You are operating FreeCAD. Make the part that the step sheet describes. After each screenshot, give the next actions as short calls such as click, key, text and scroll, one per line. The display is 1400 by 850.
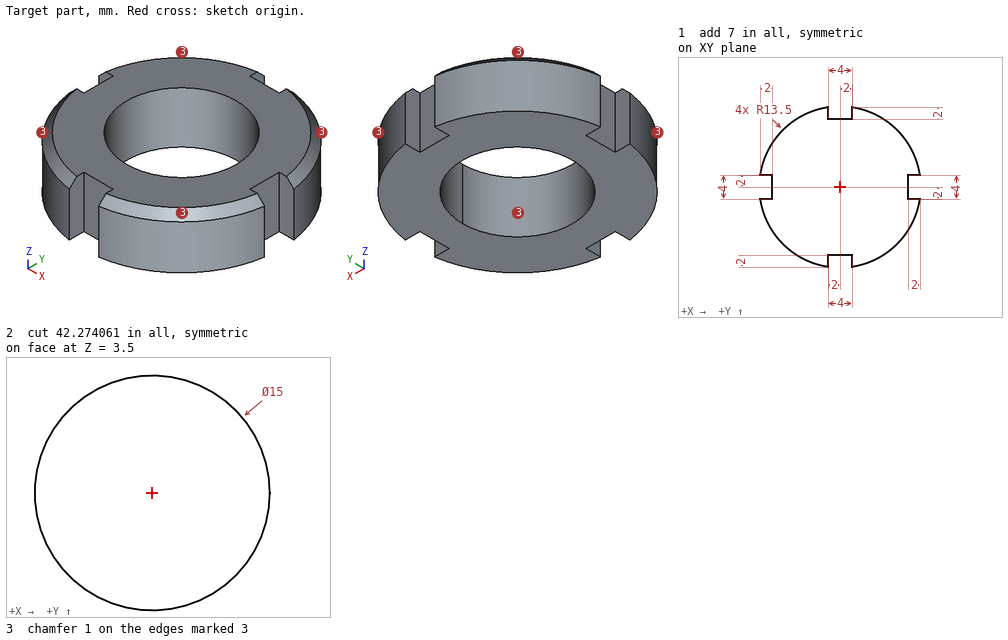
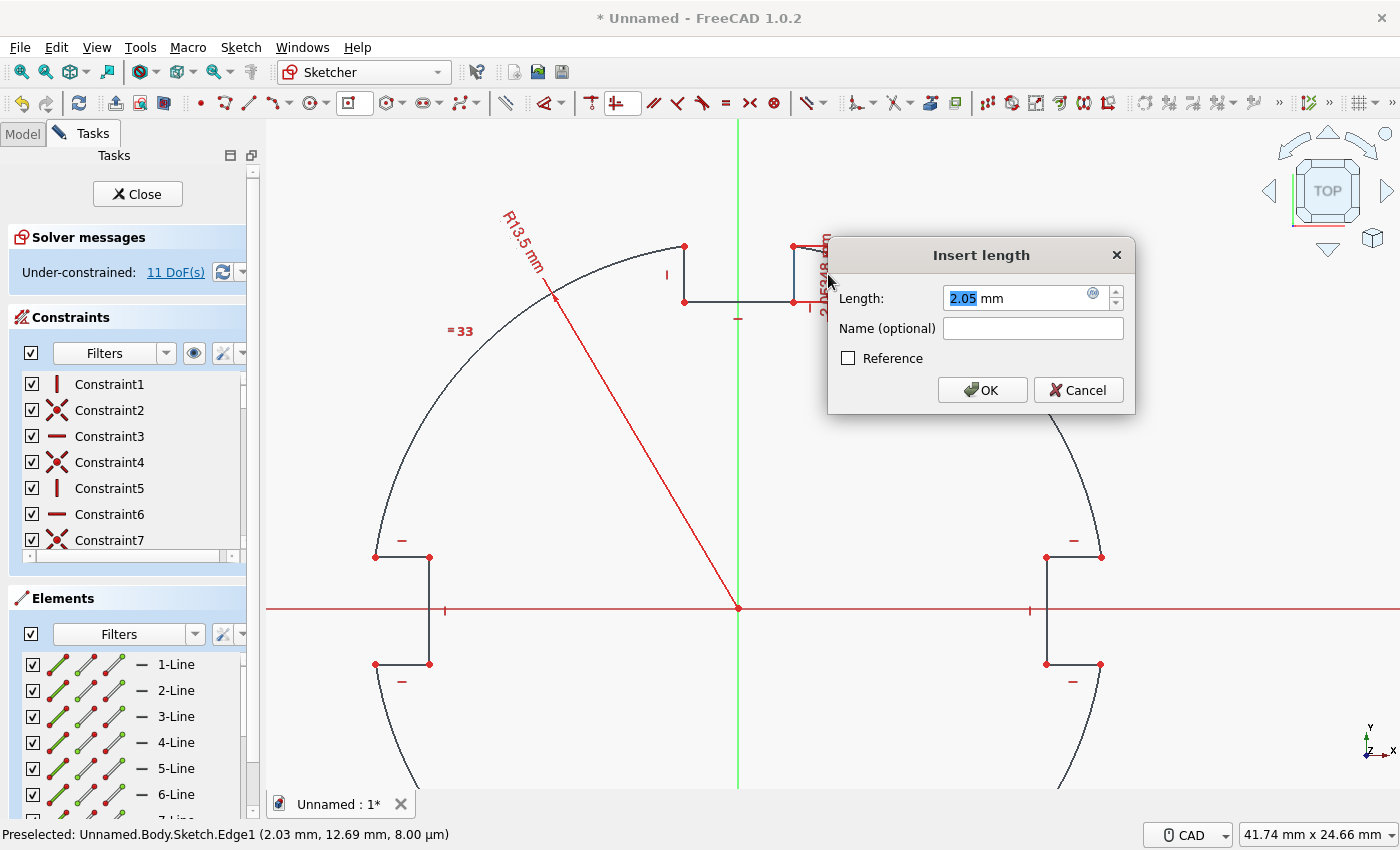
text(2)
key(Return)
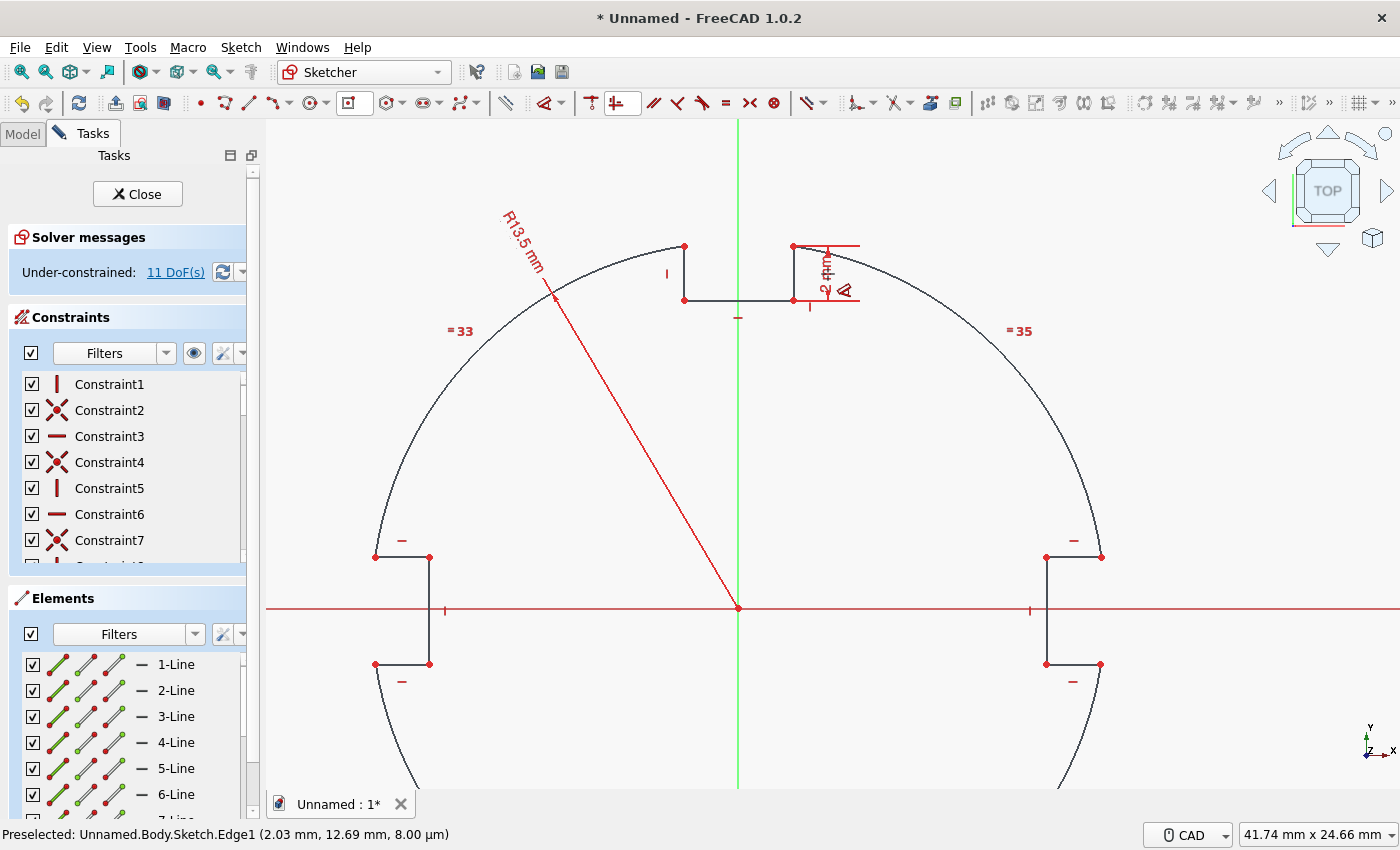
click(761, 301)
click(714, 267)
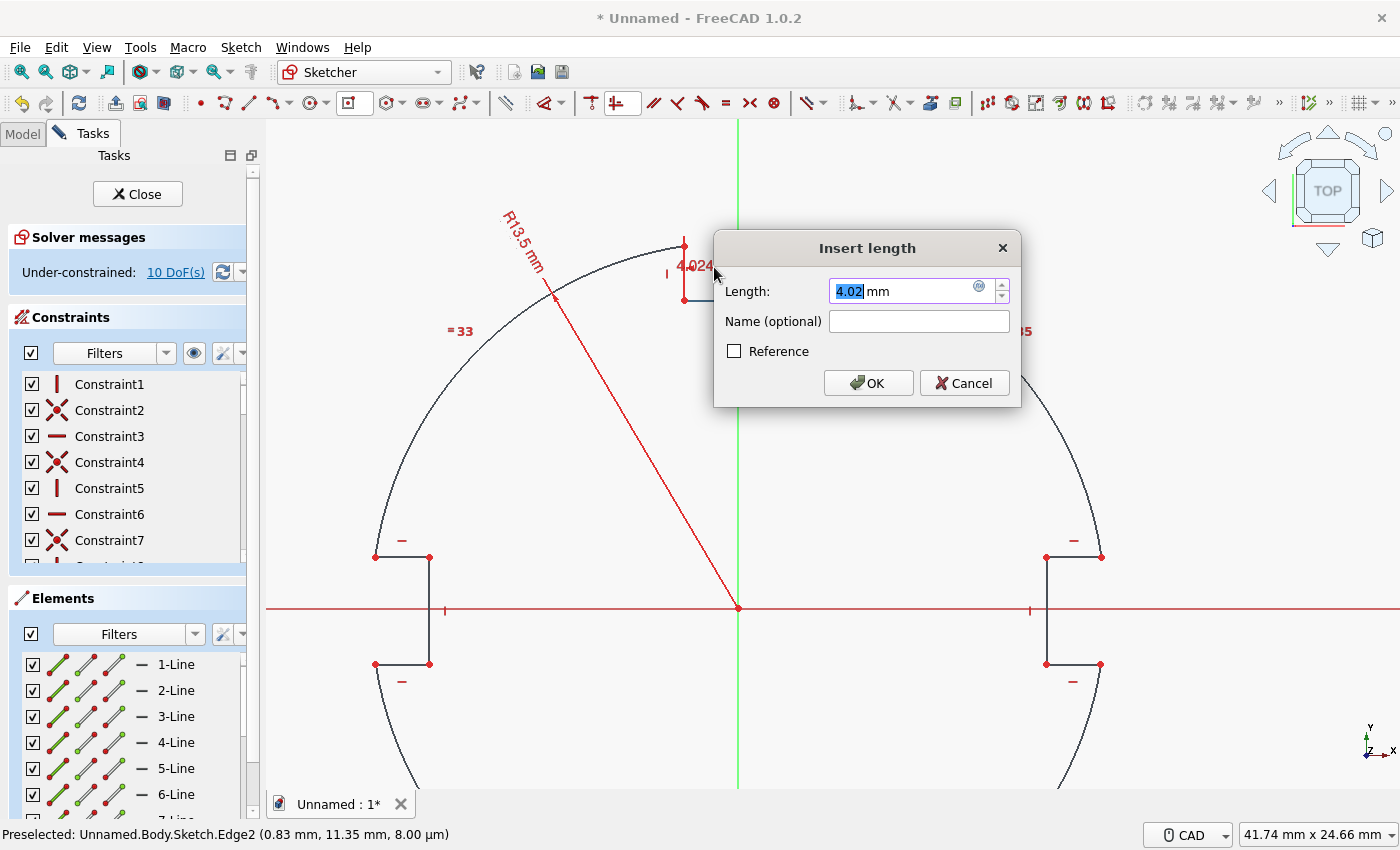
text(4)
key(Return)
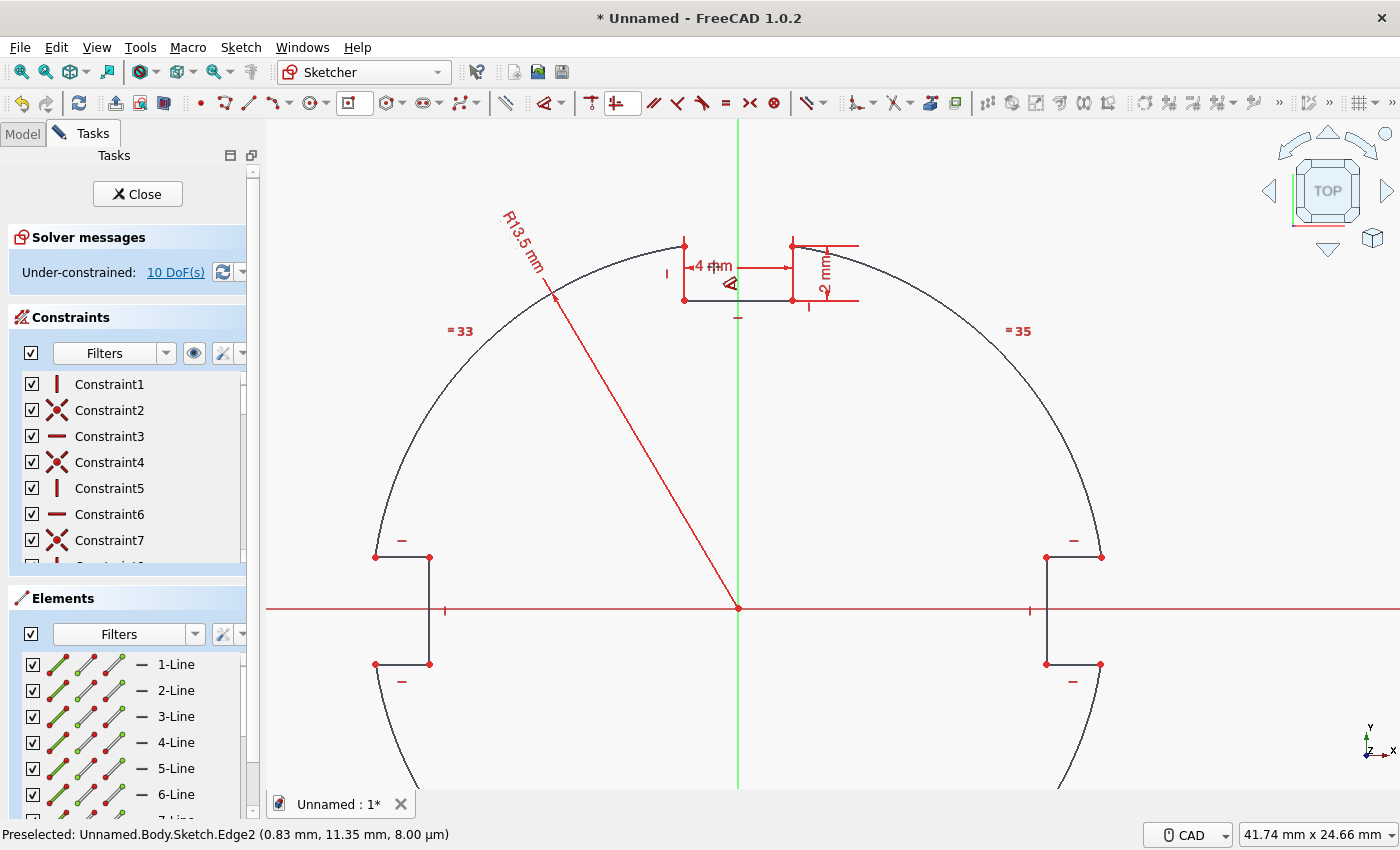
click(391, 557)
click(402, 523)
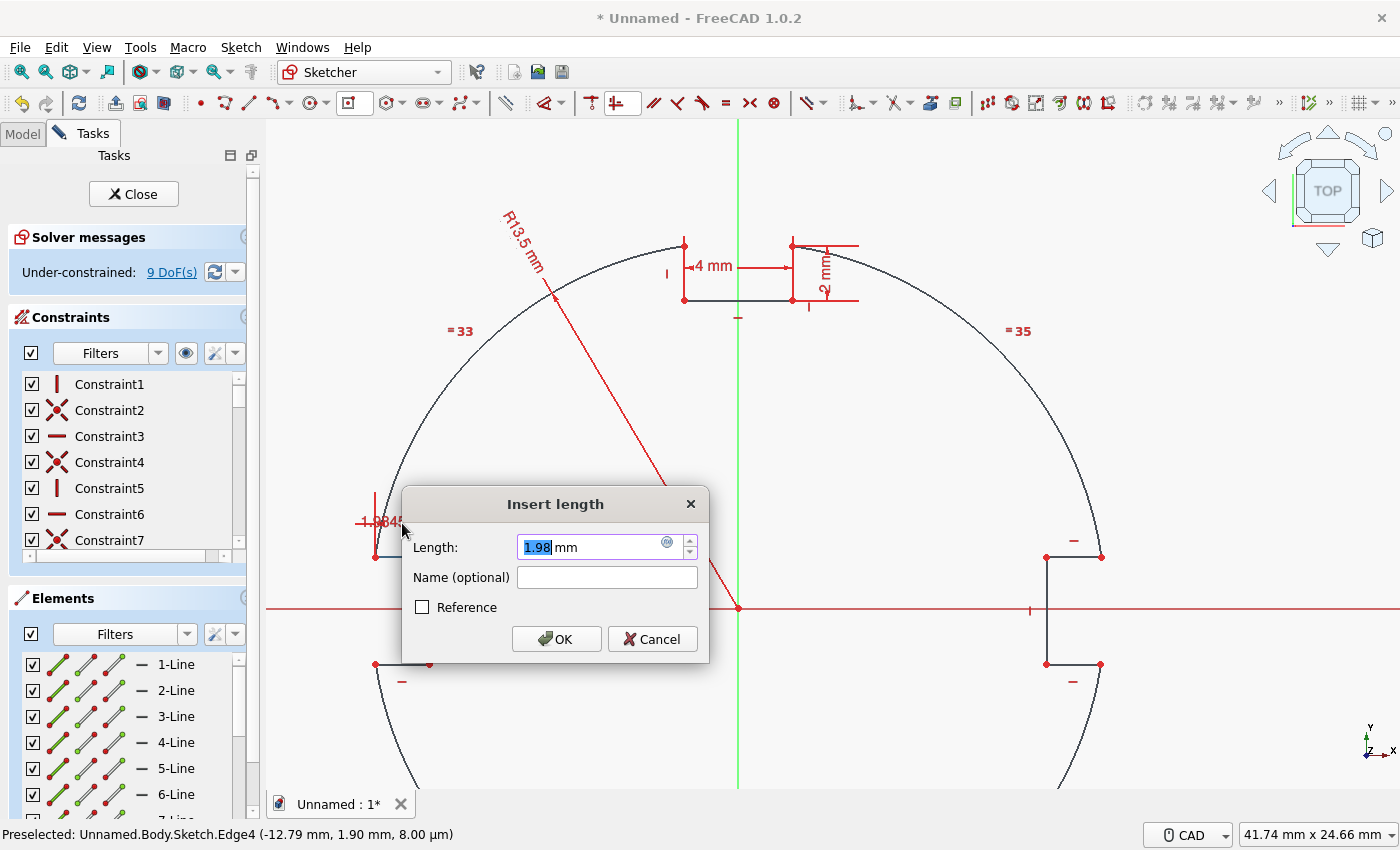
text(2)
key(Return)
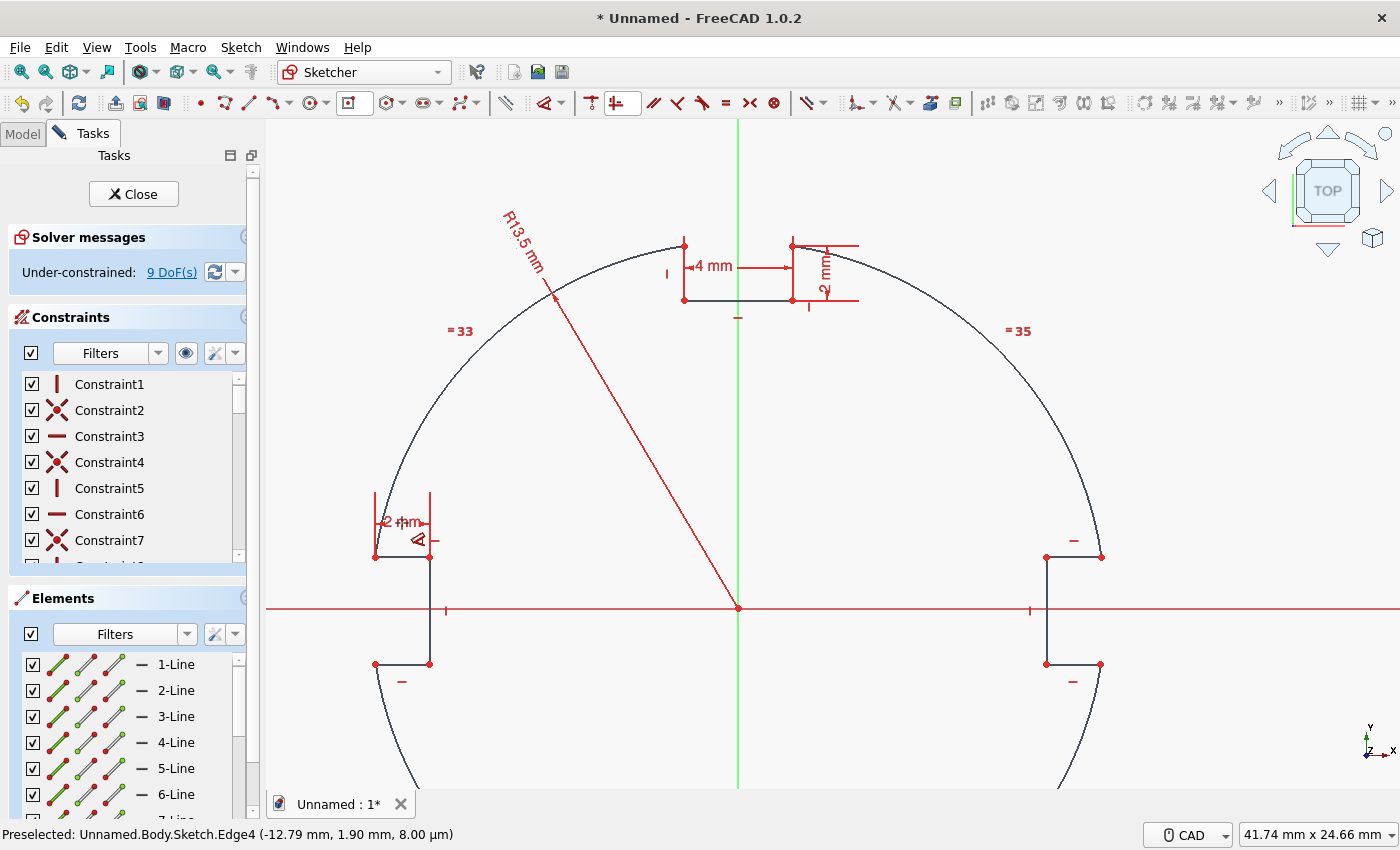
click(430, 589)
click(396, 586)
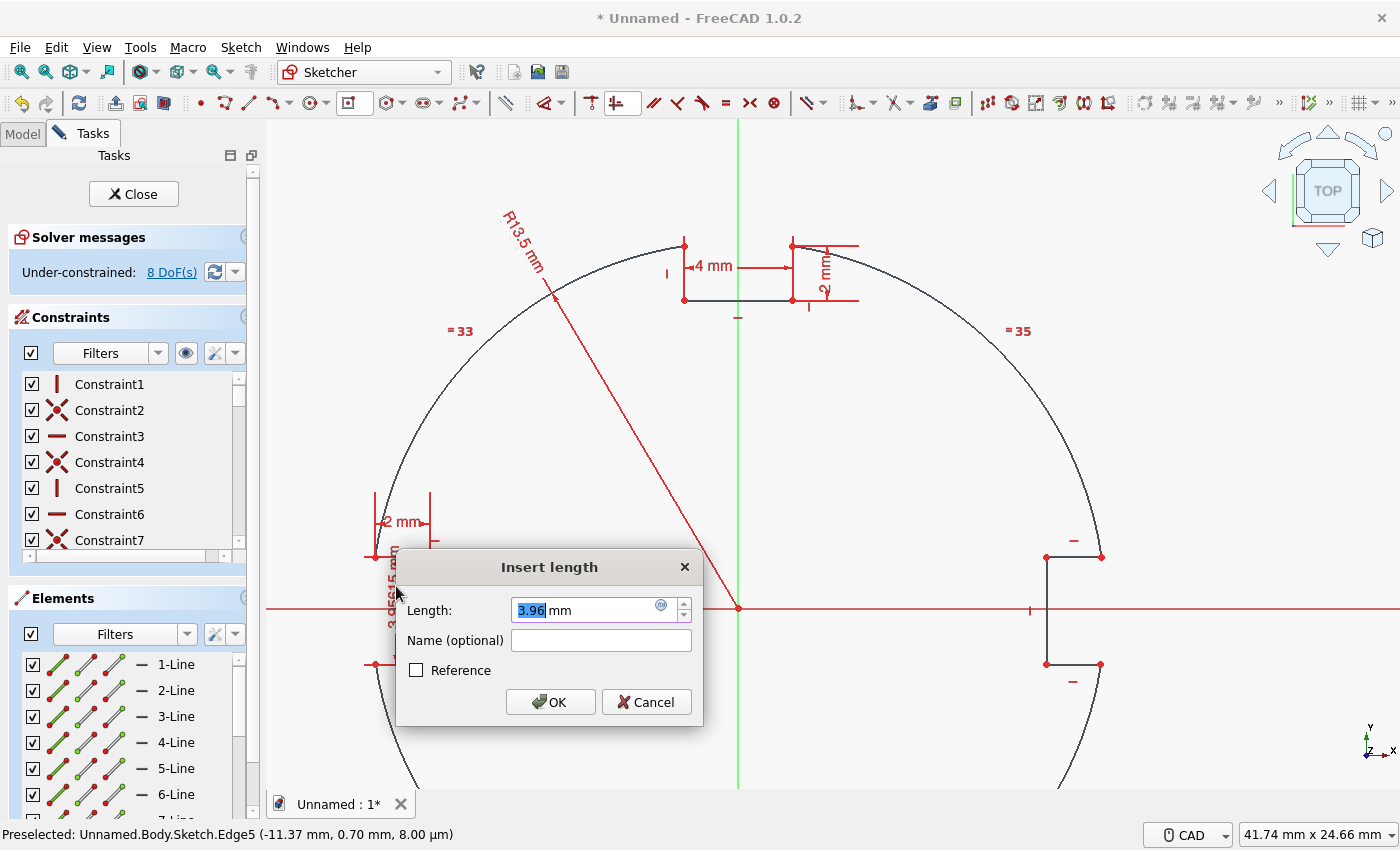
text(4)
key(Return)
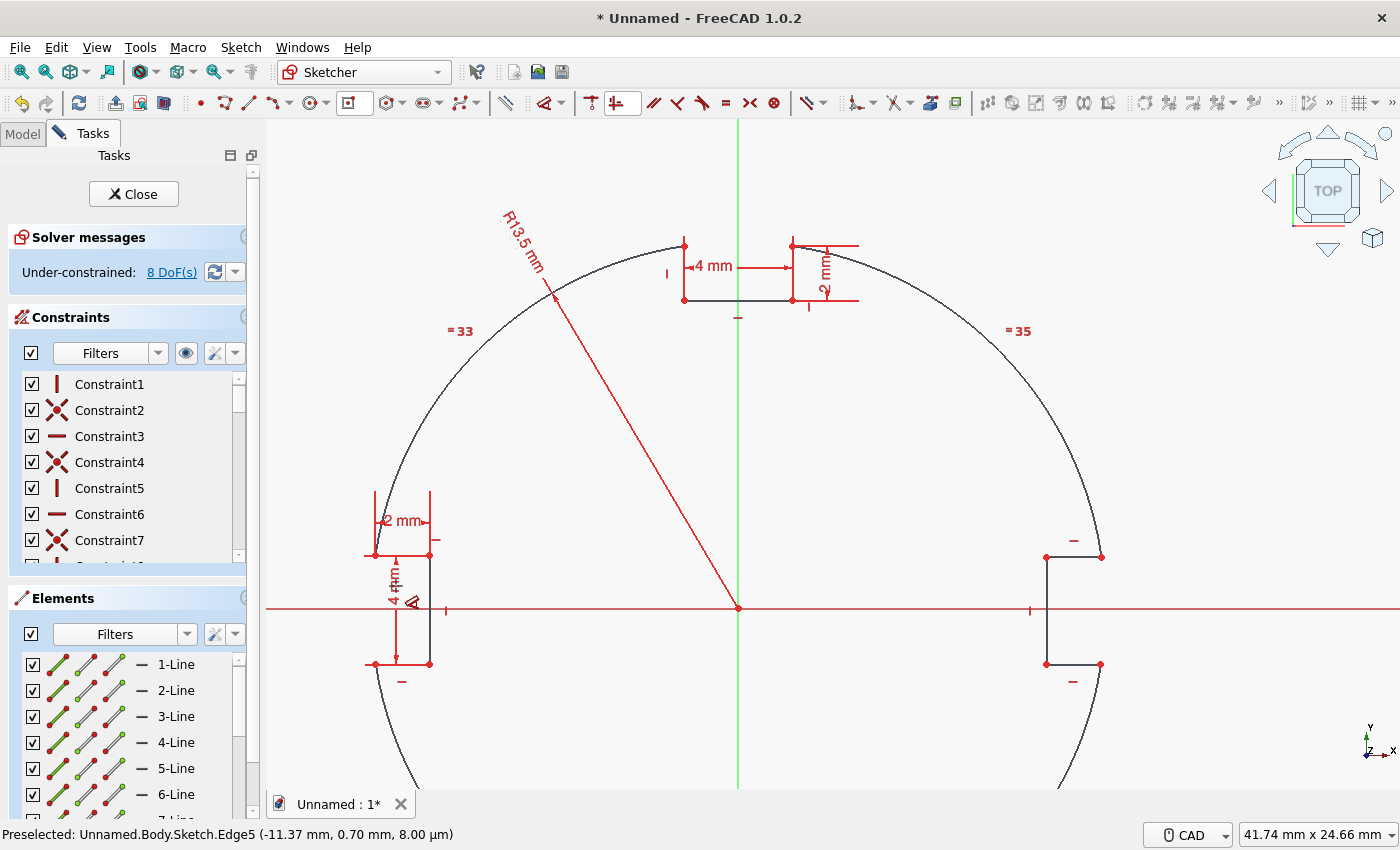
scroll(796, 266, down, 3)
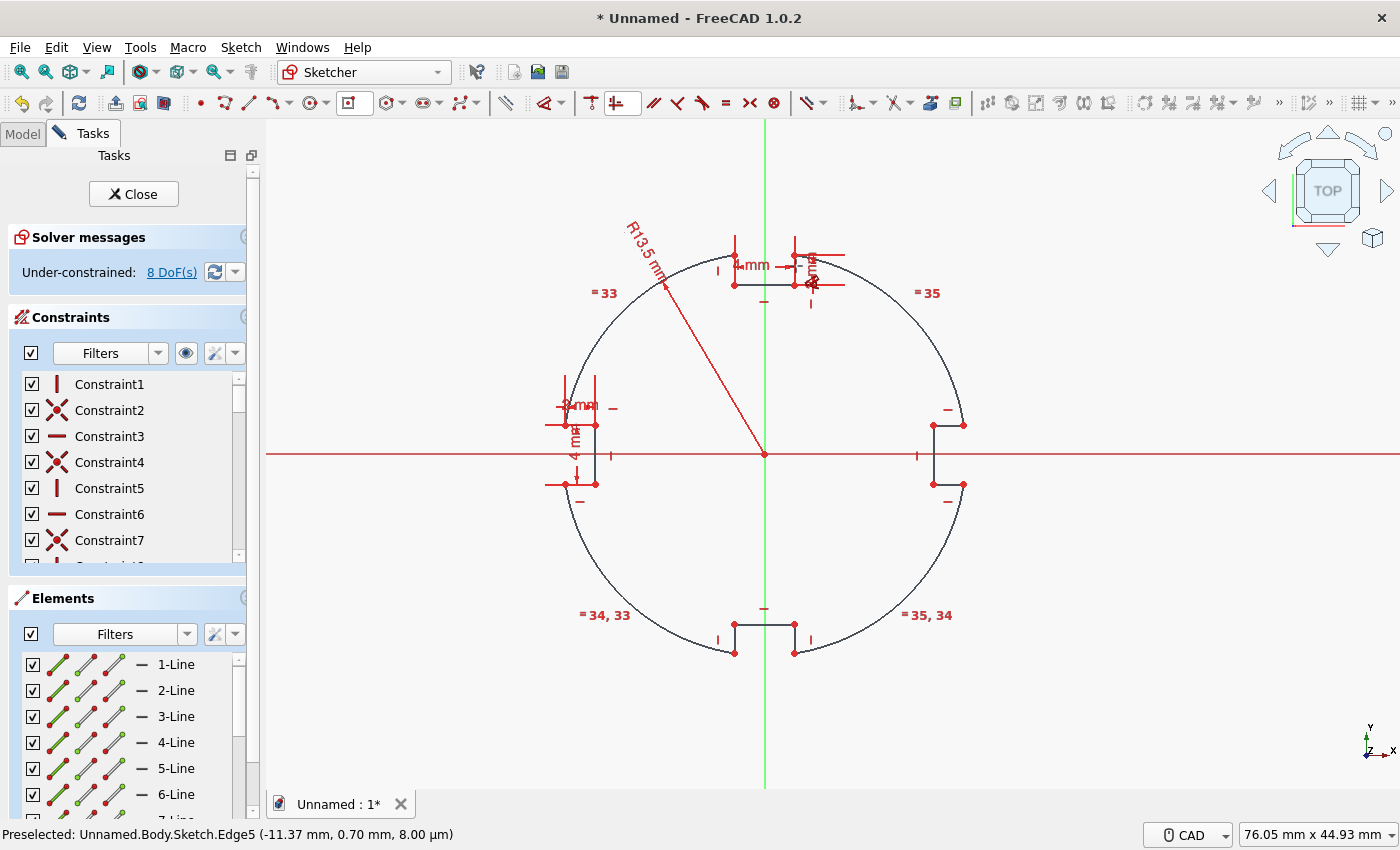
scroll(735, 645, up, 3)